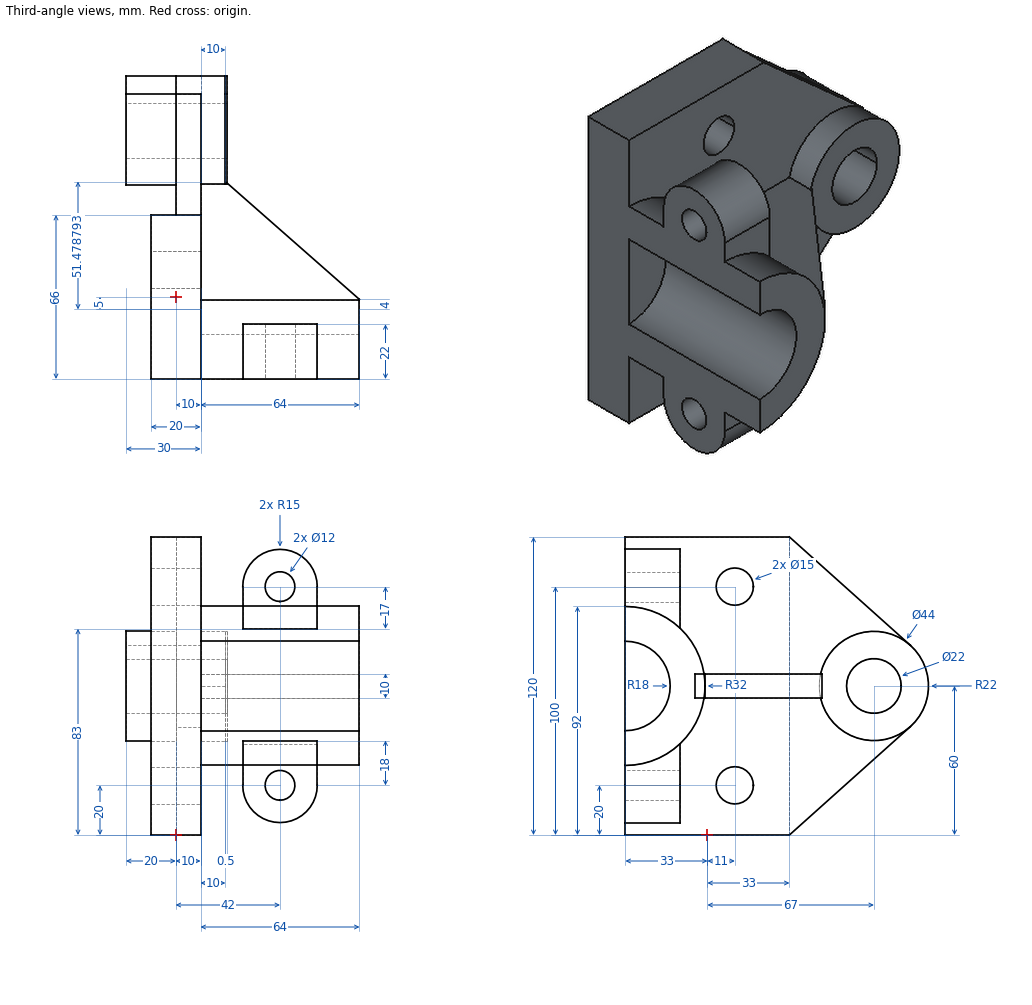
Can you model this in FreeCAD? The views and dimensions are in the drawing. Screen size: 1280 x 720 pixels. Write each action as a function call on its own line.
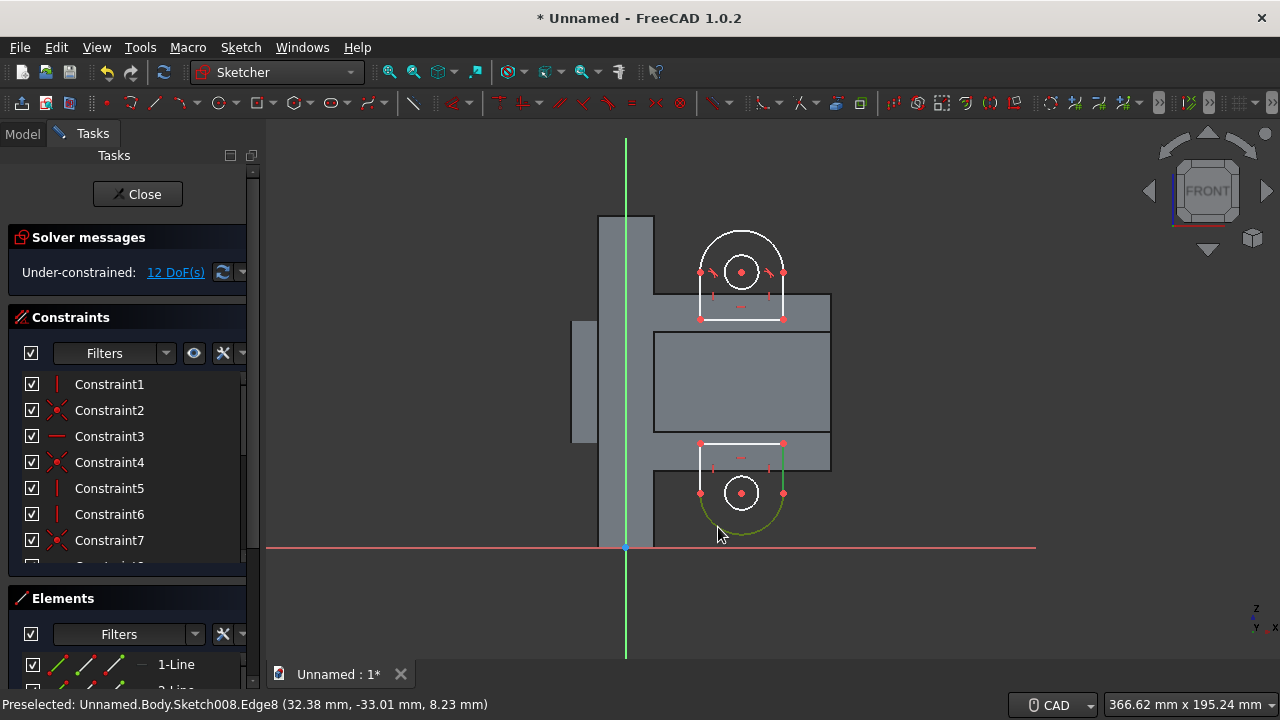
click(608, 104)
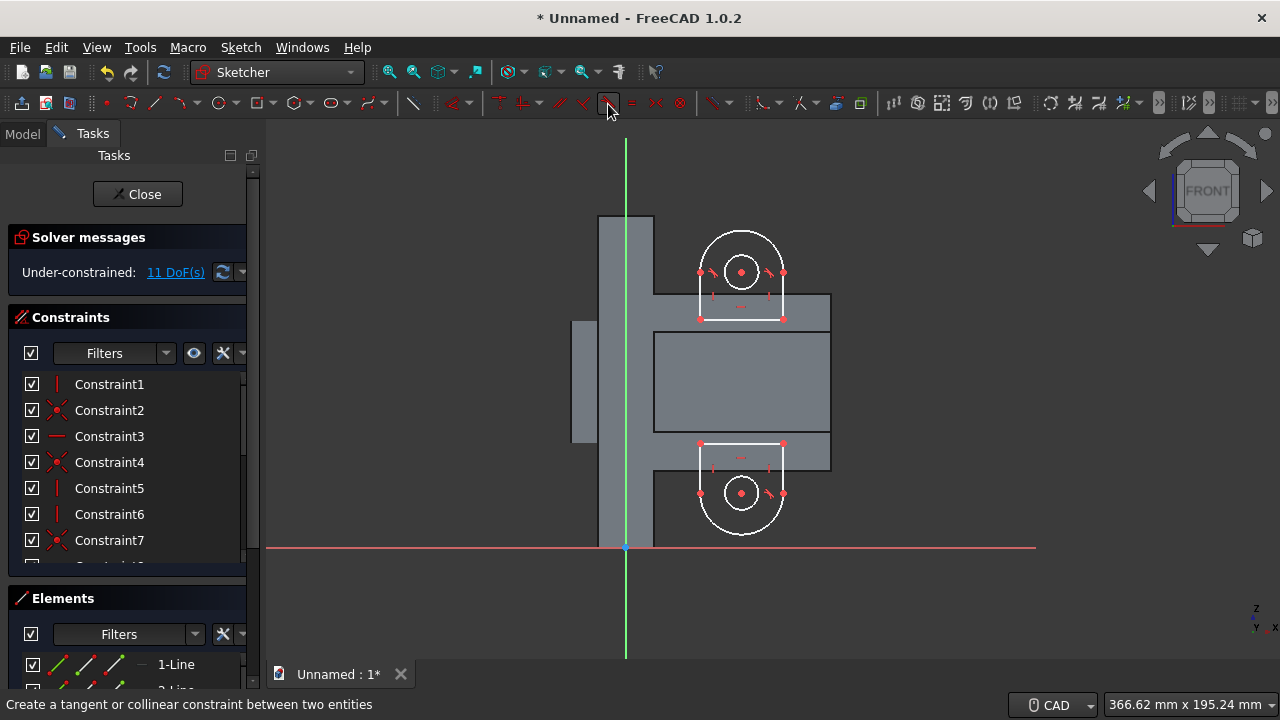
click(700, 459)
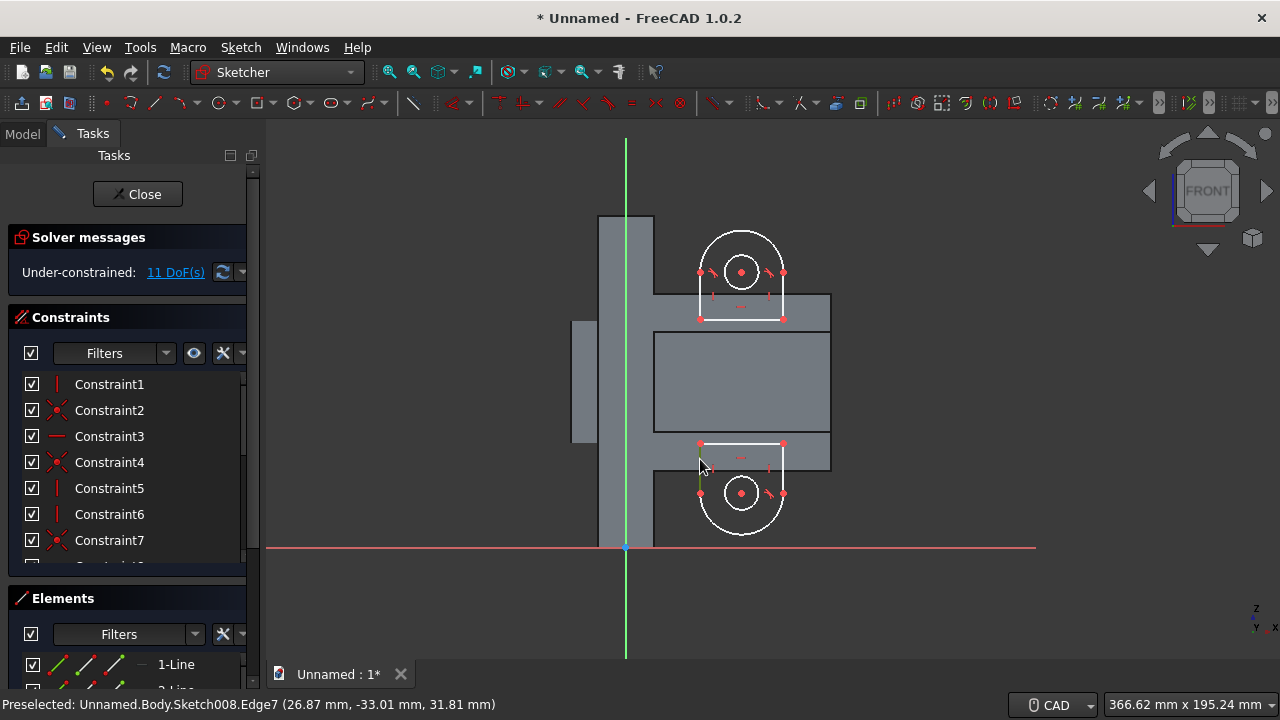
click(718, 527)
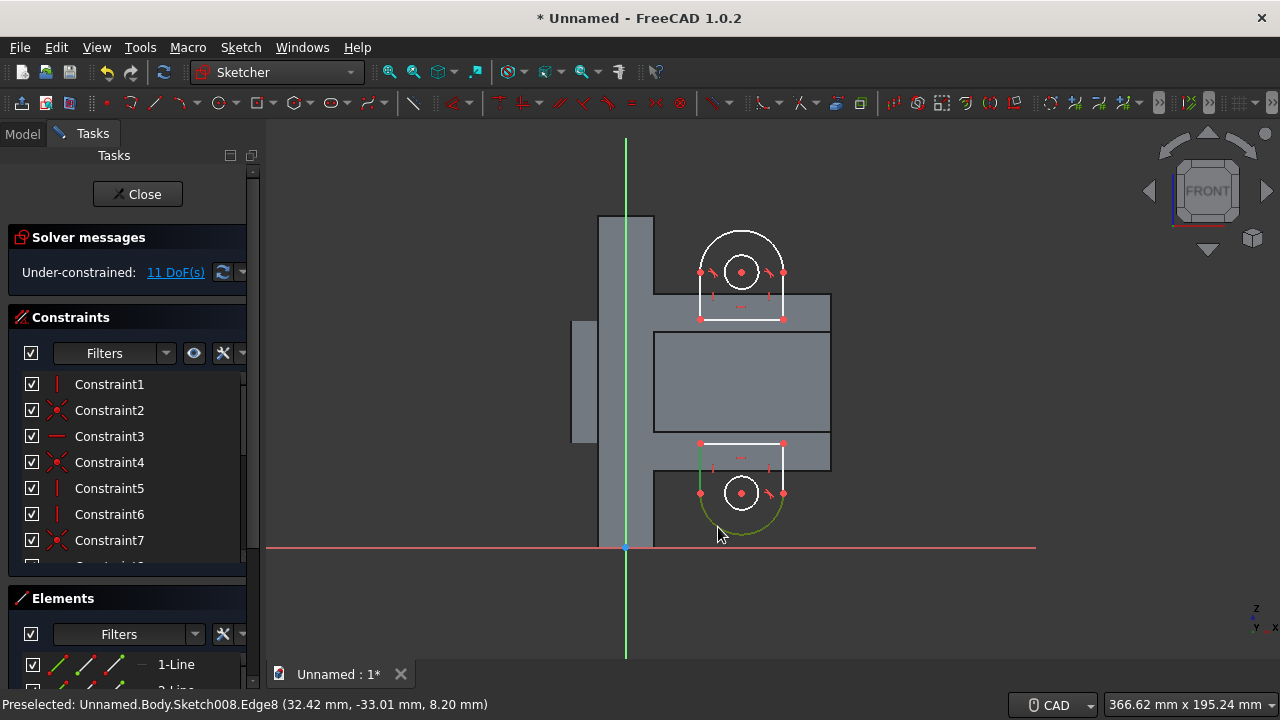
click(608, 104)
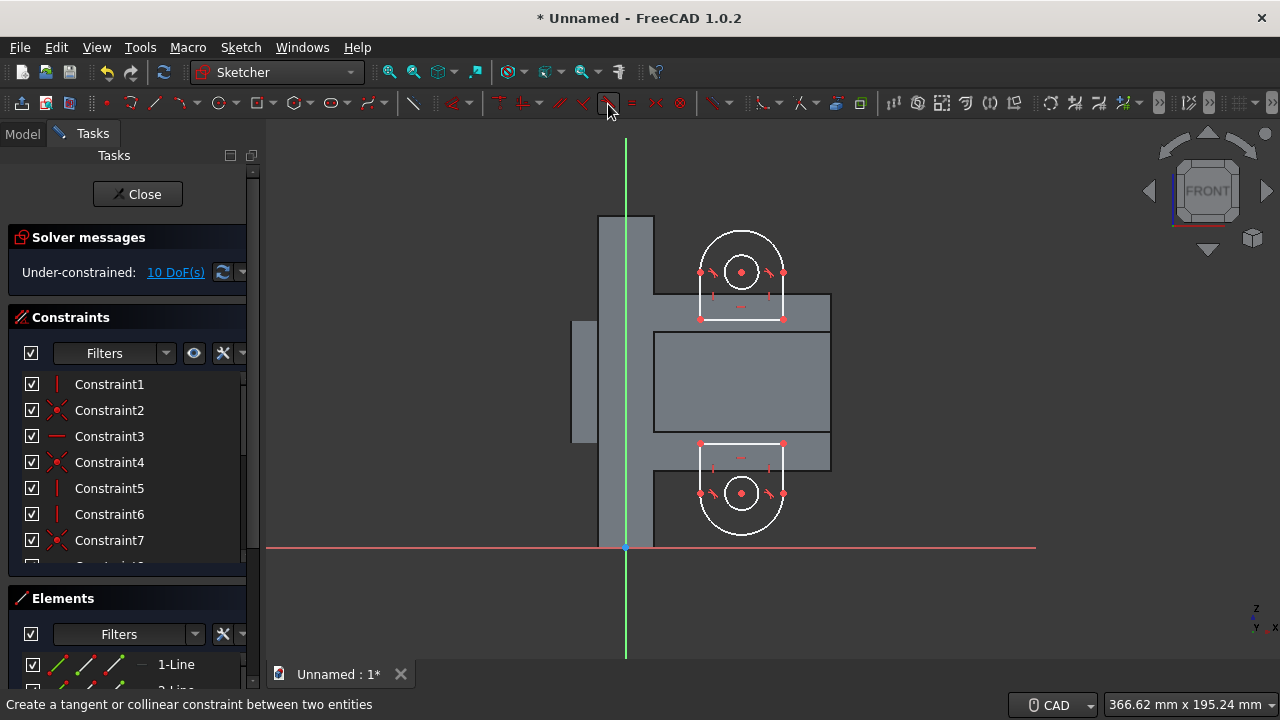
click(766, 239)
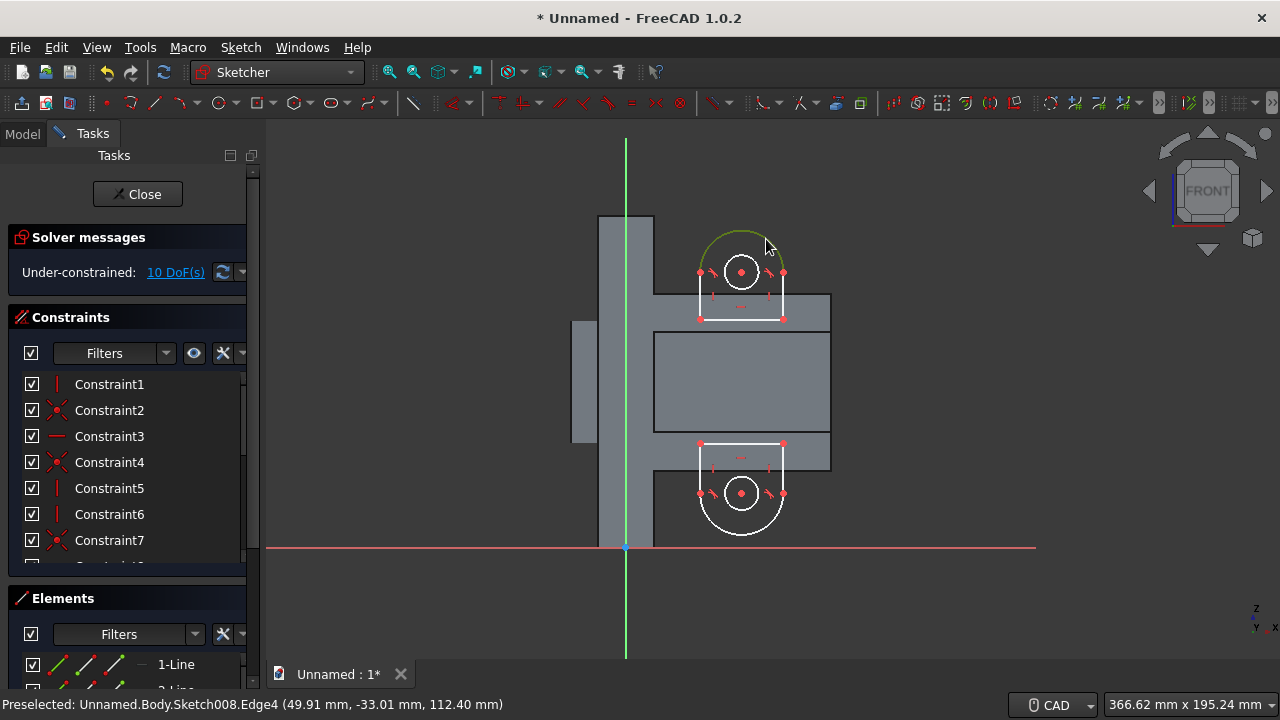
click(717, 527)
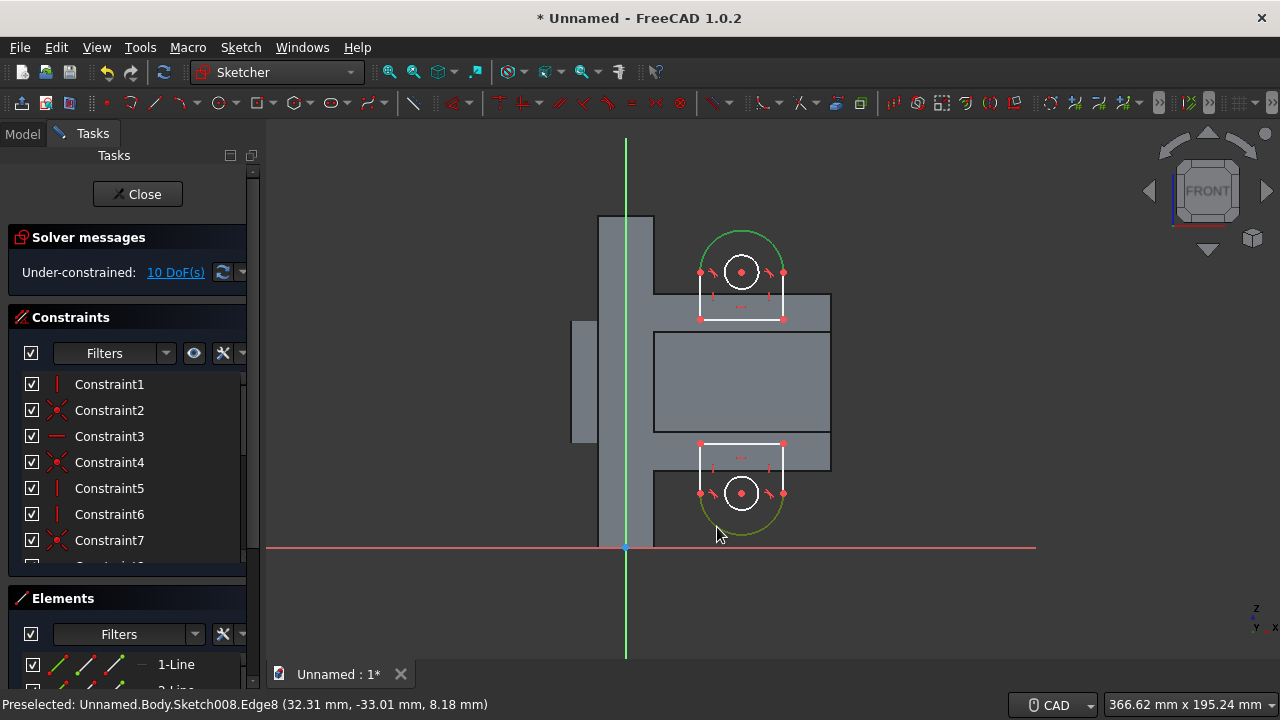
click(632, 104)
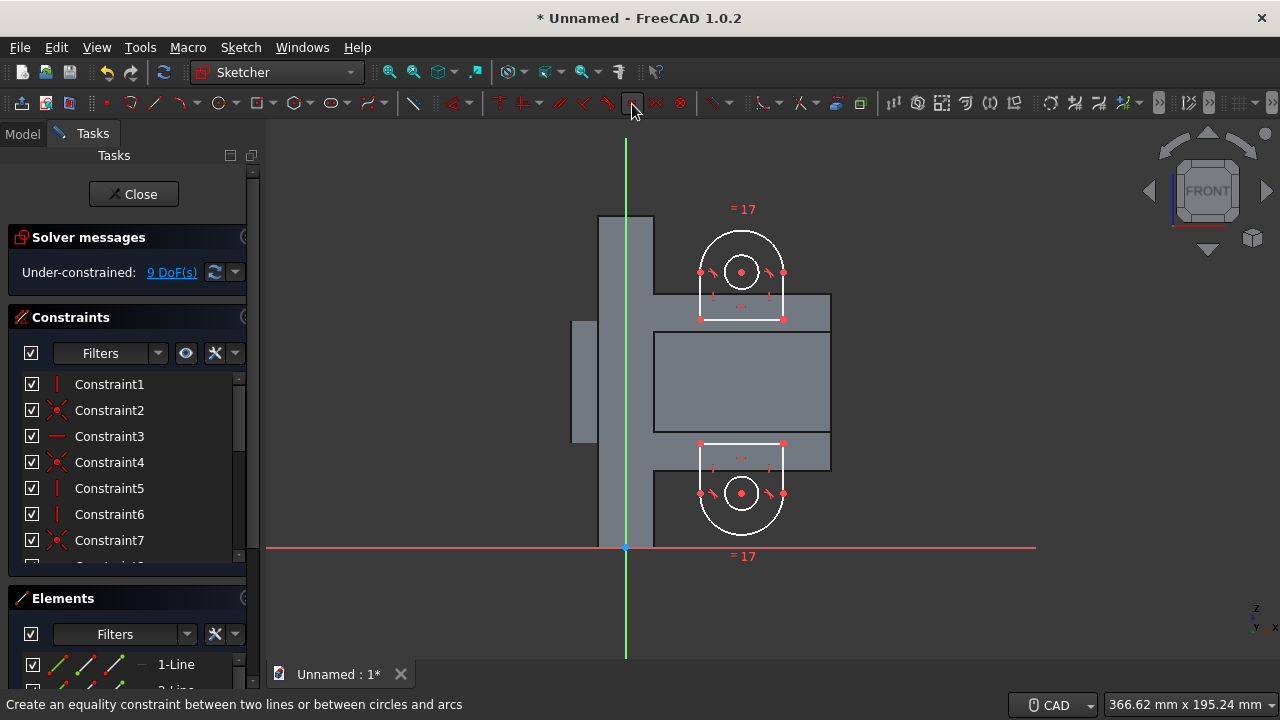
click(754, 260)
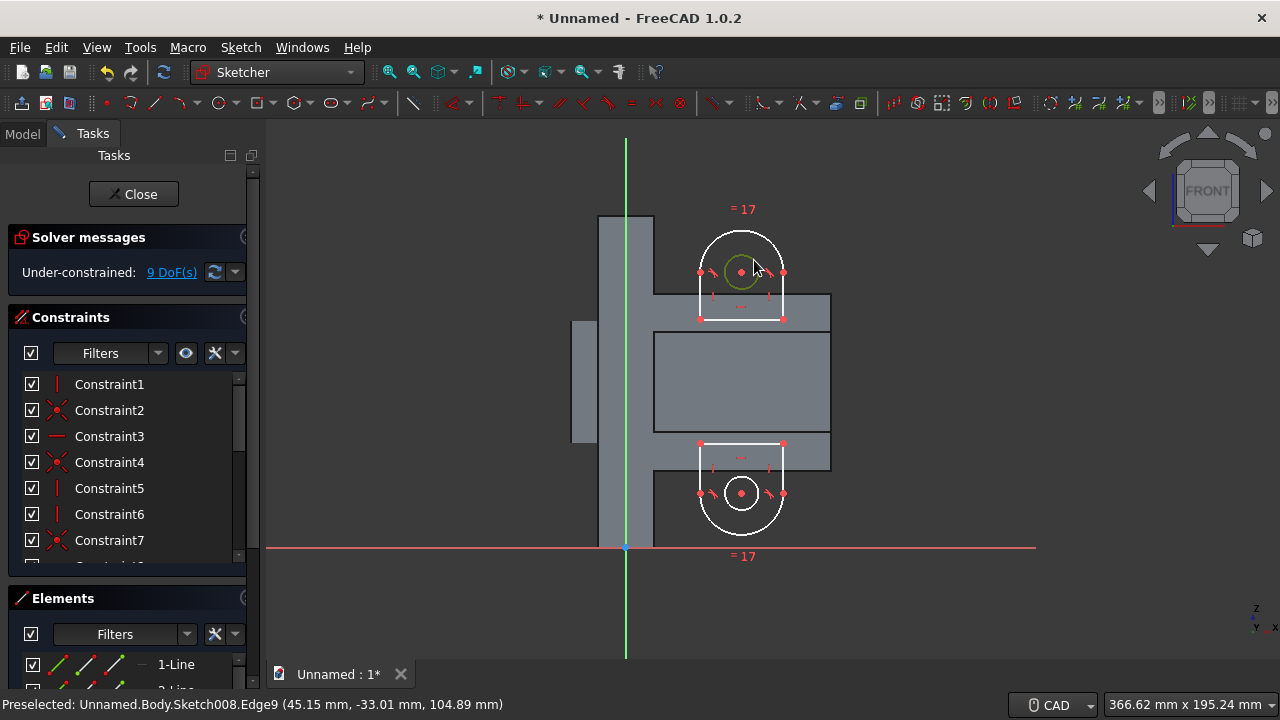
click(753, 482)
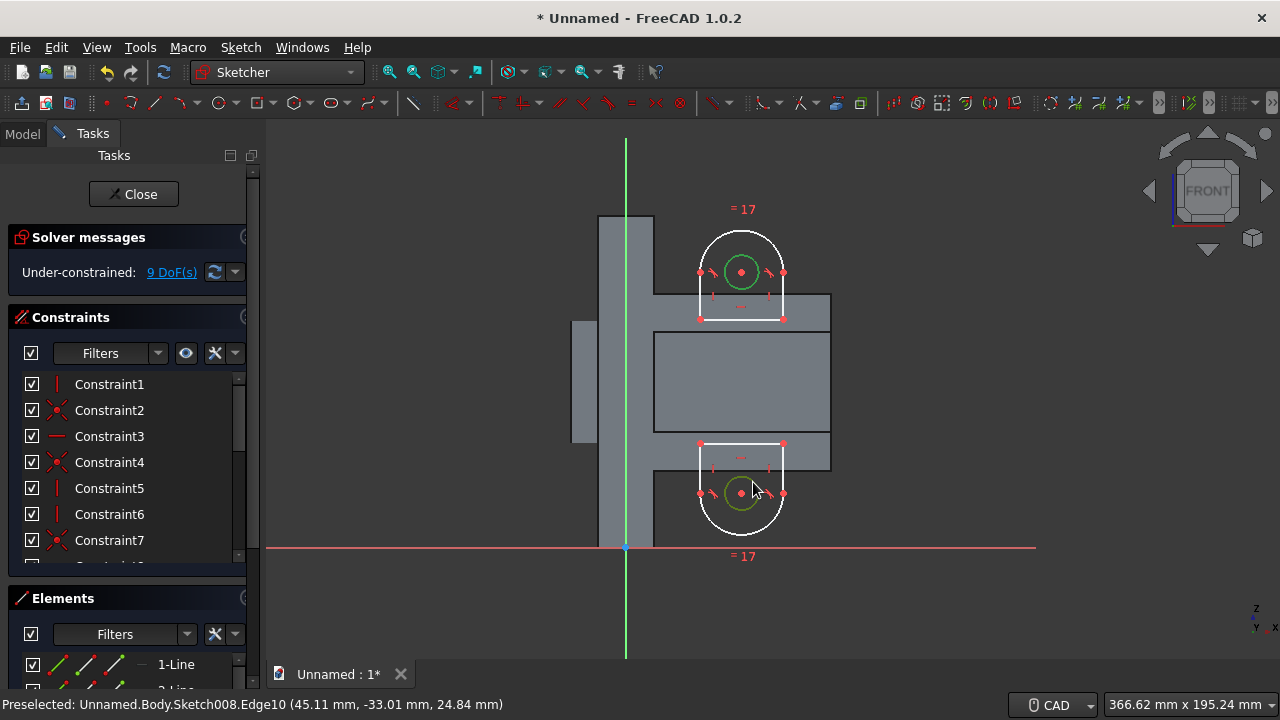
click(632, 104)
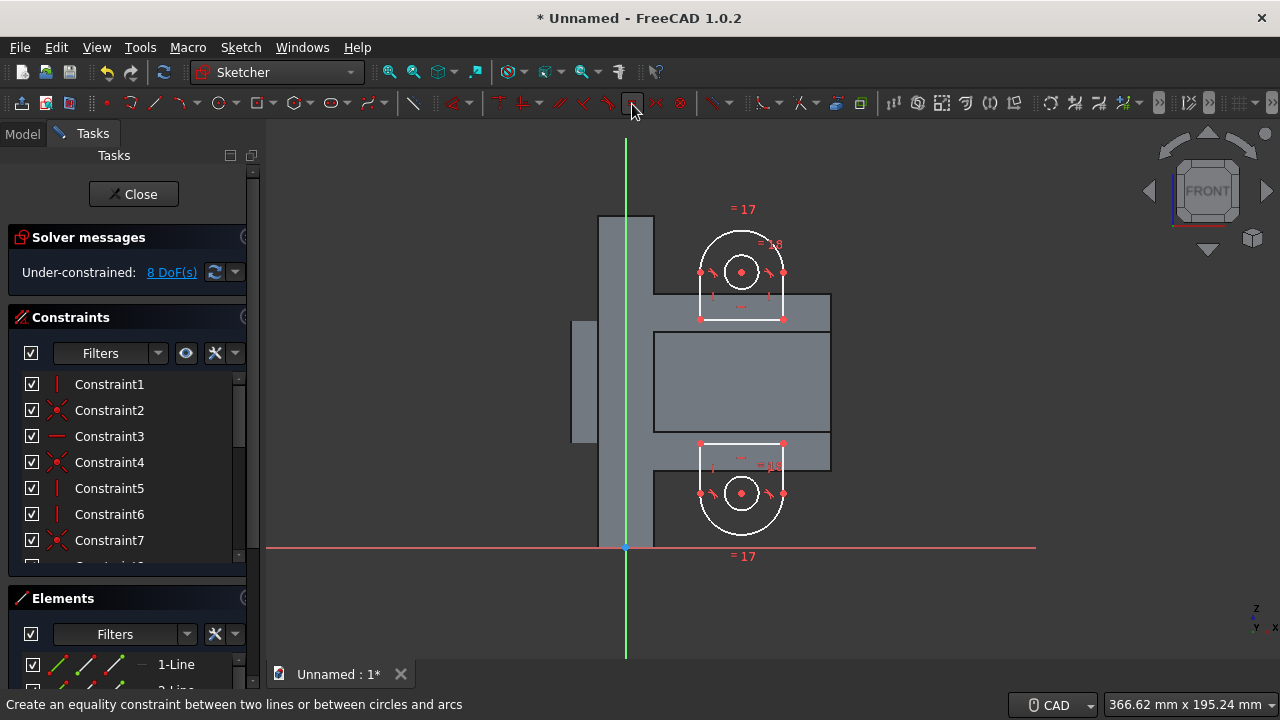
click(452, 104)